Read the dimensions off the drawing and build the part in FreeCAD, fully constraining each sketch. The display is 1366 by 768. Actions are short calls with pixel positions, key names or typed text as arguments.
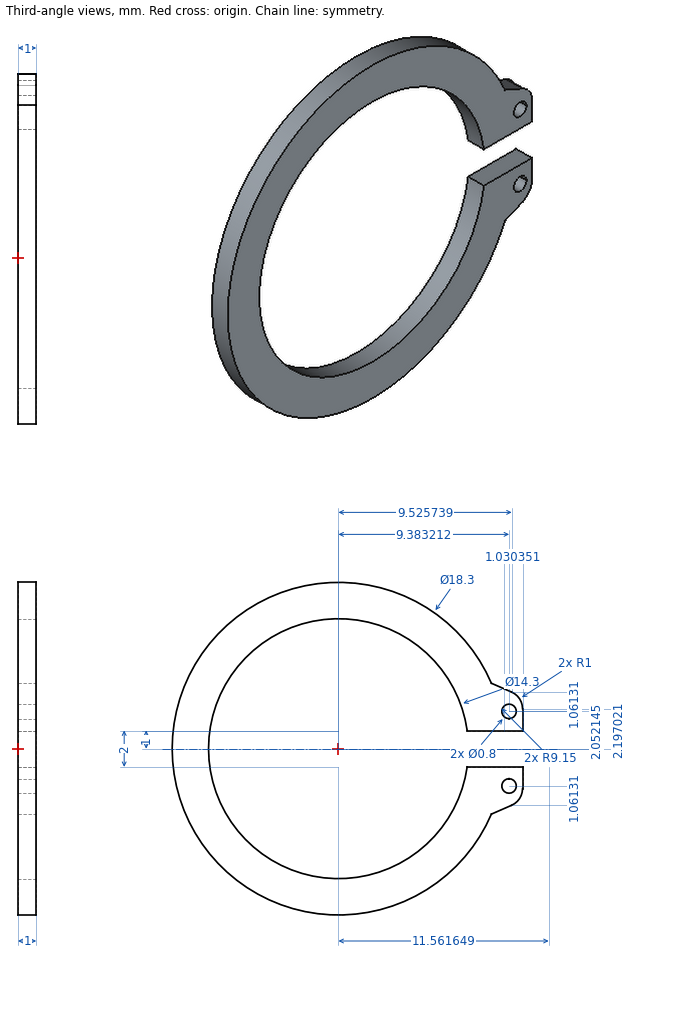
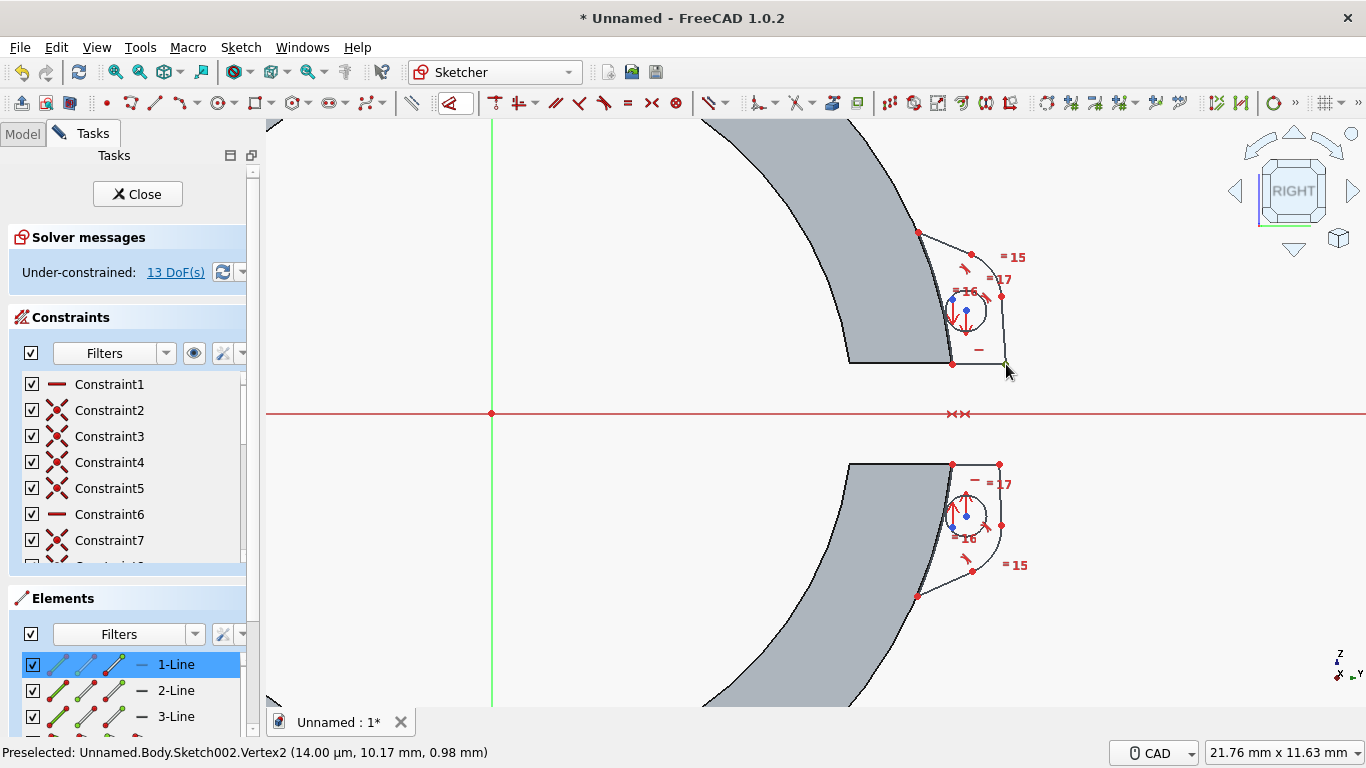
click(999, 465)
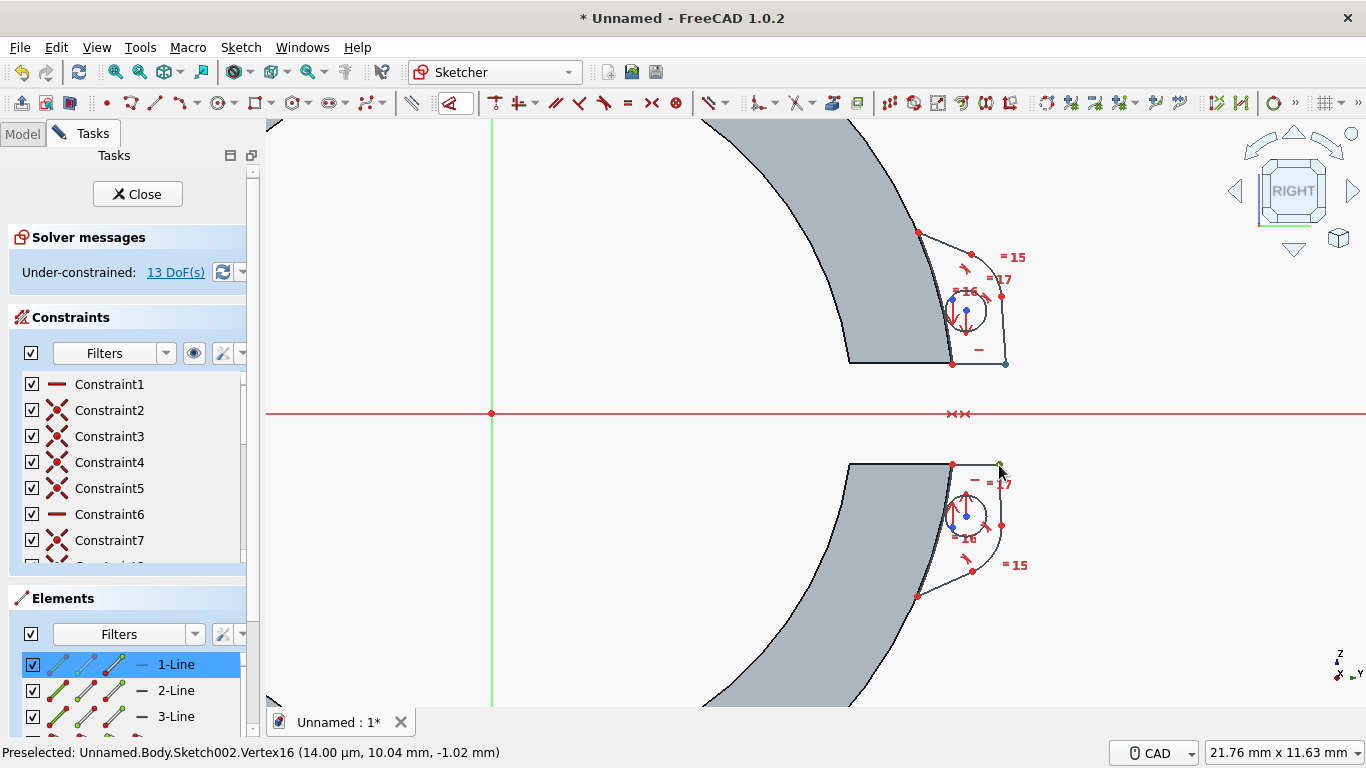
click(359, 414)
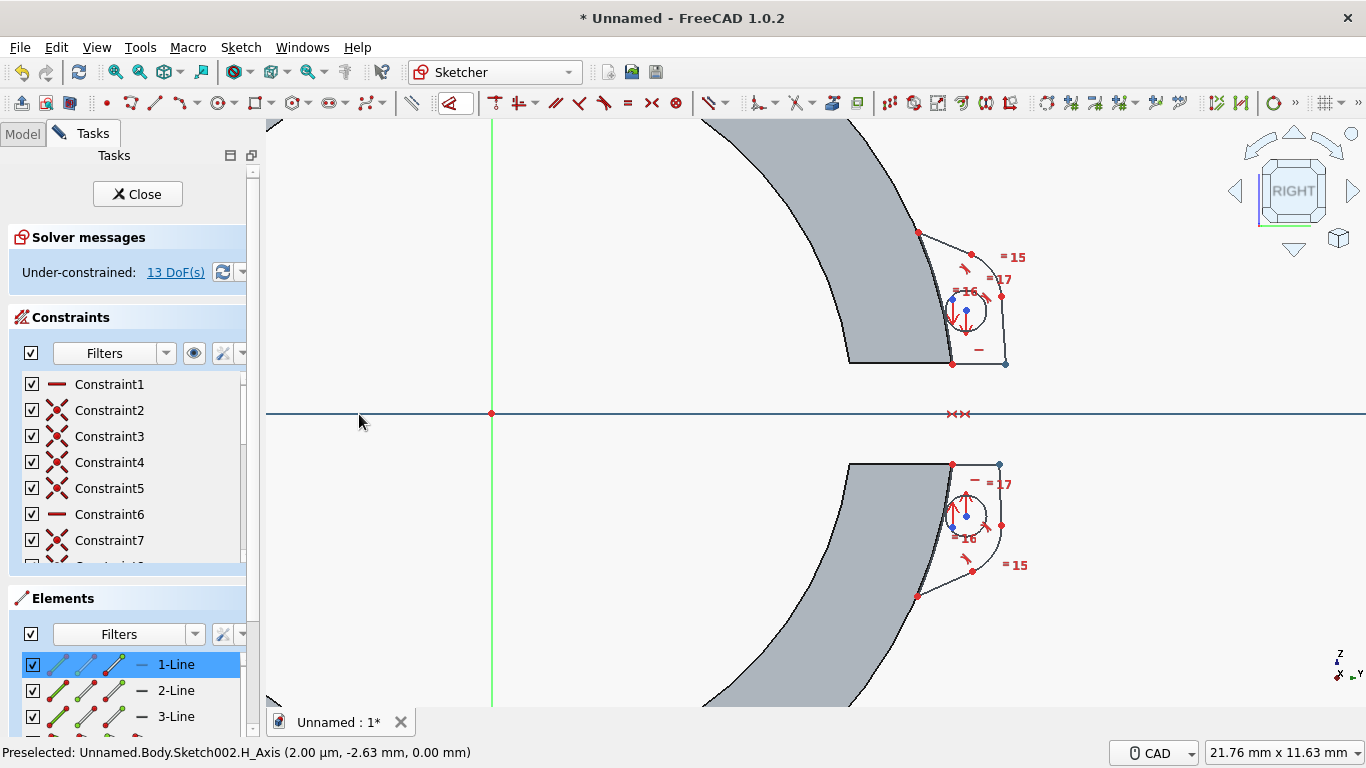
click(652, 104)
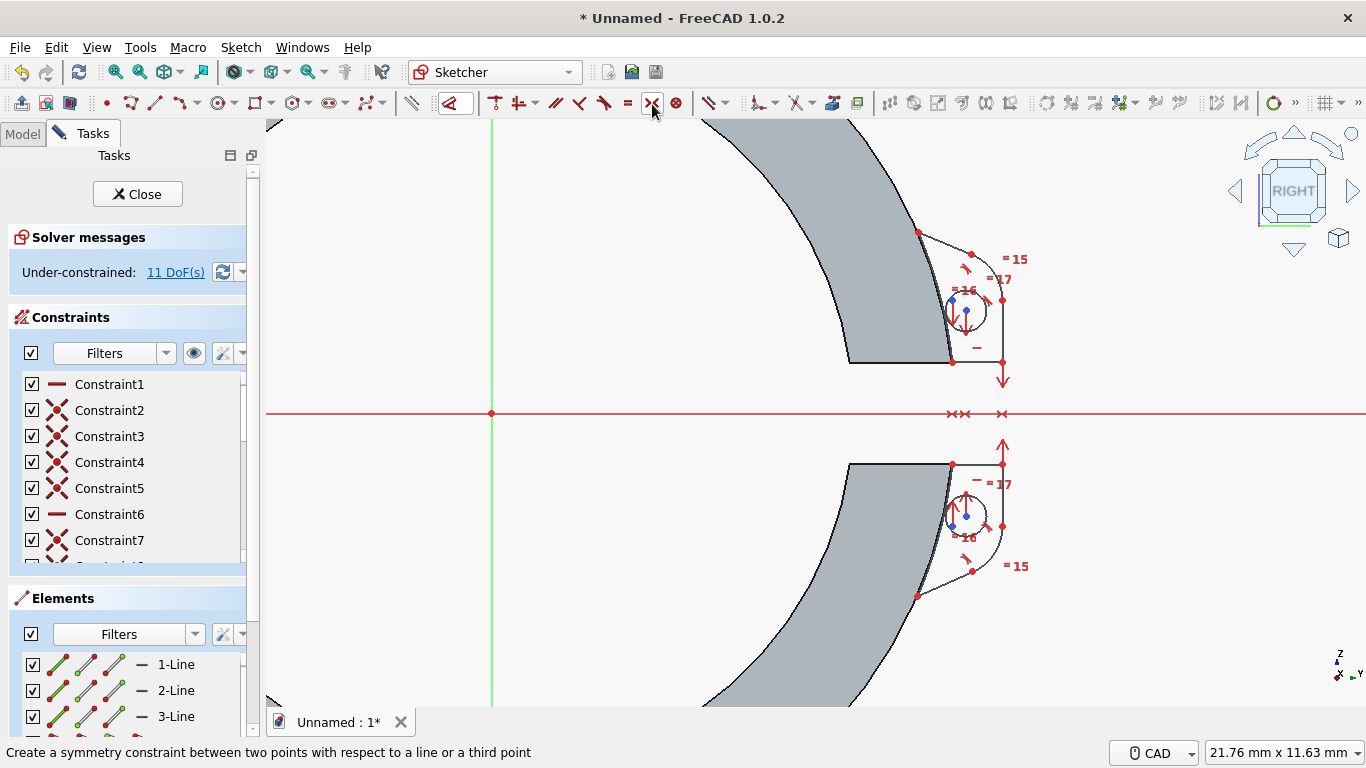
click(987, 264)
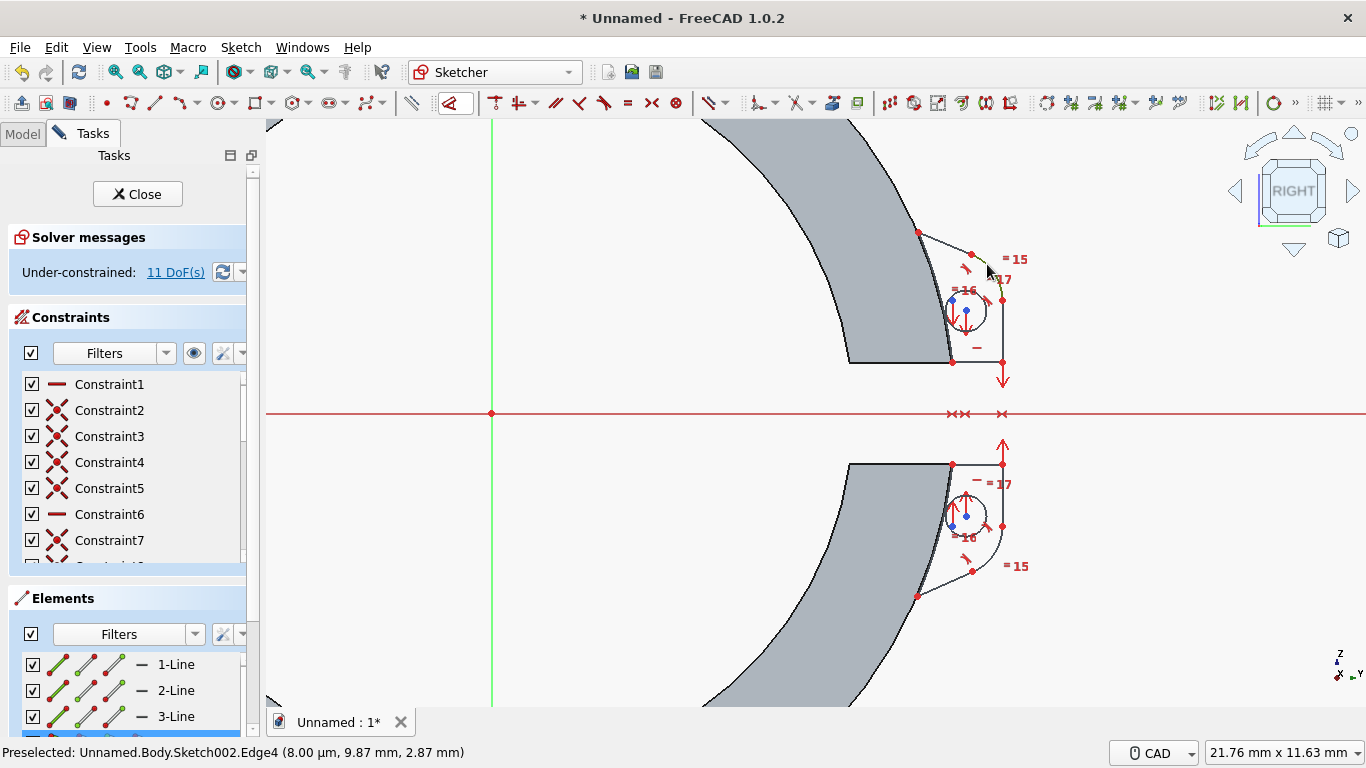
click(468, 104)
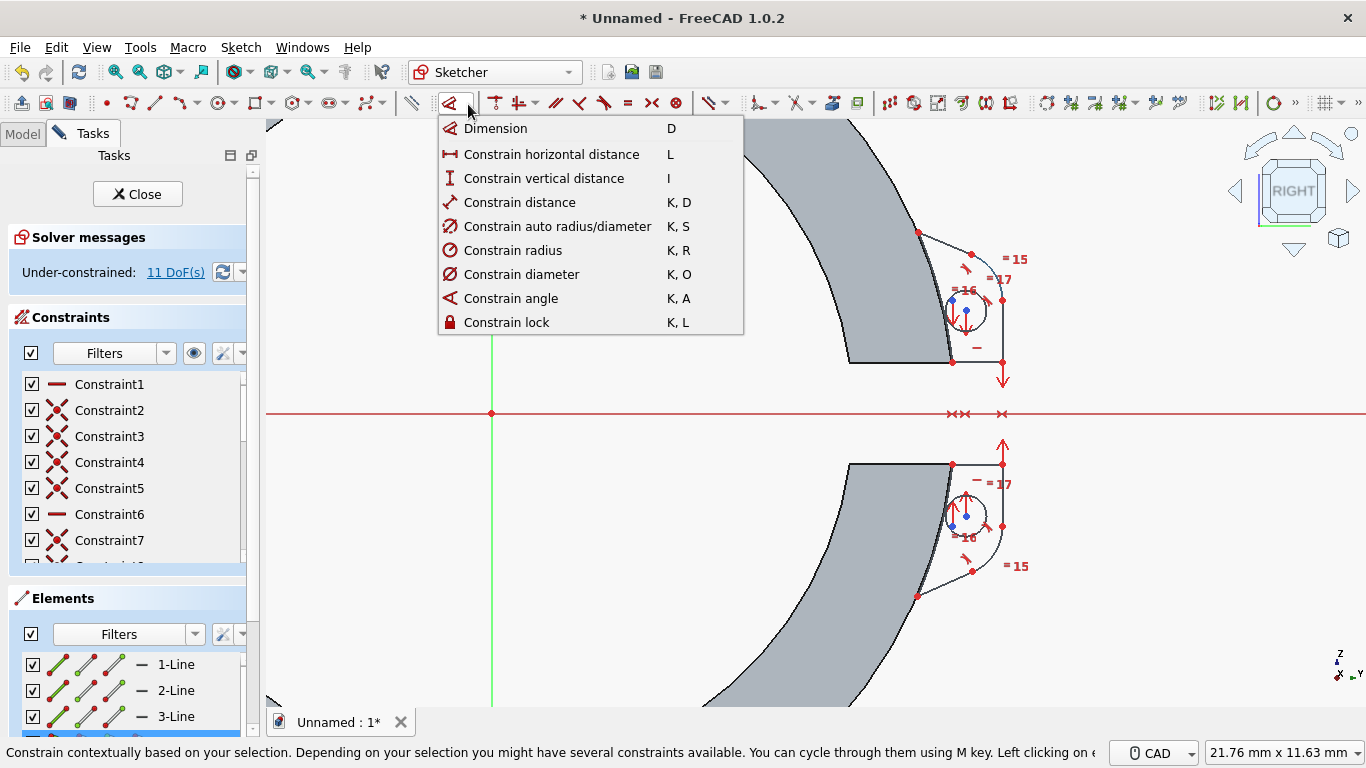
click(591, 250)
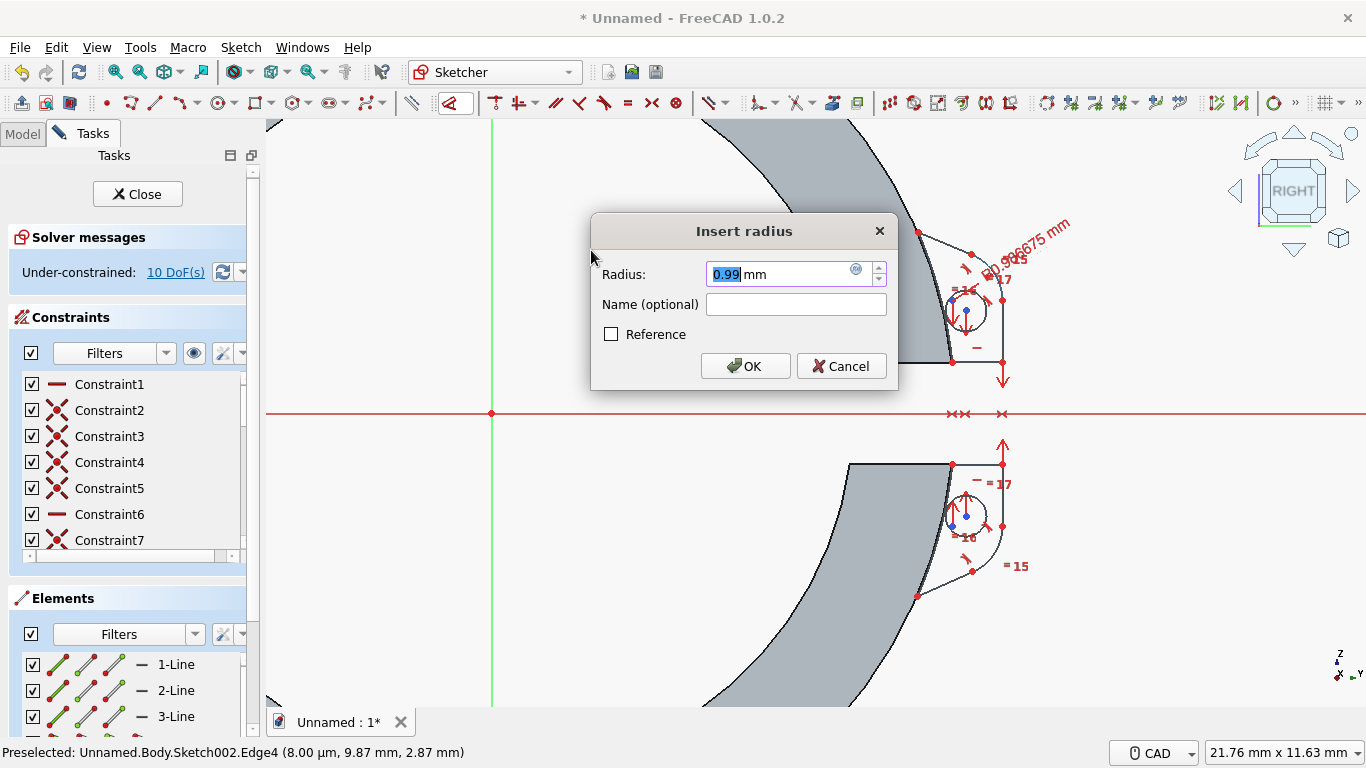
text(1)
key(Return)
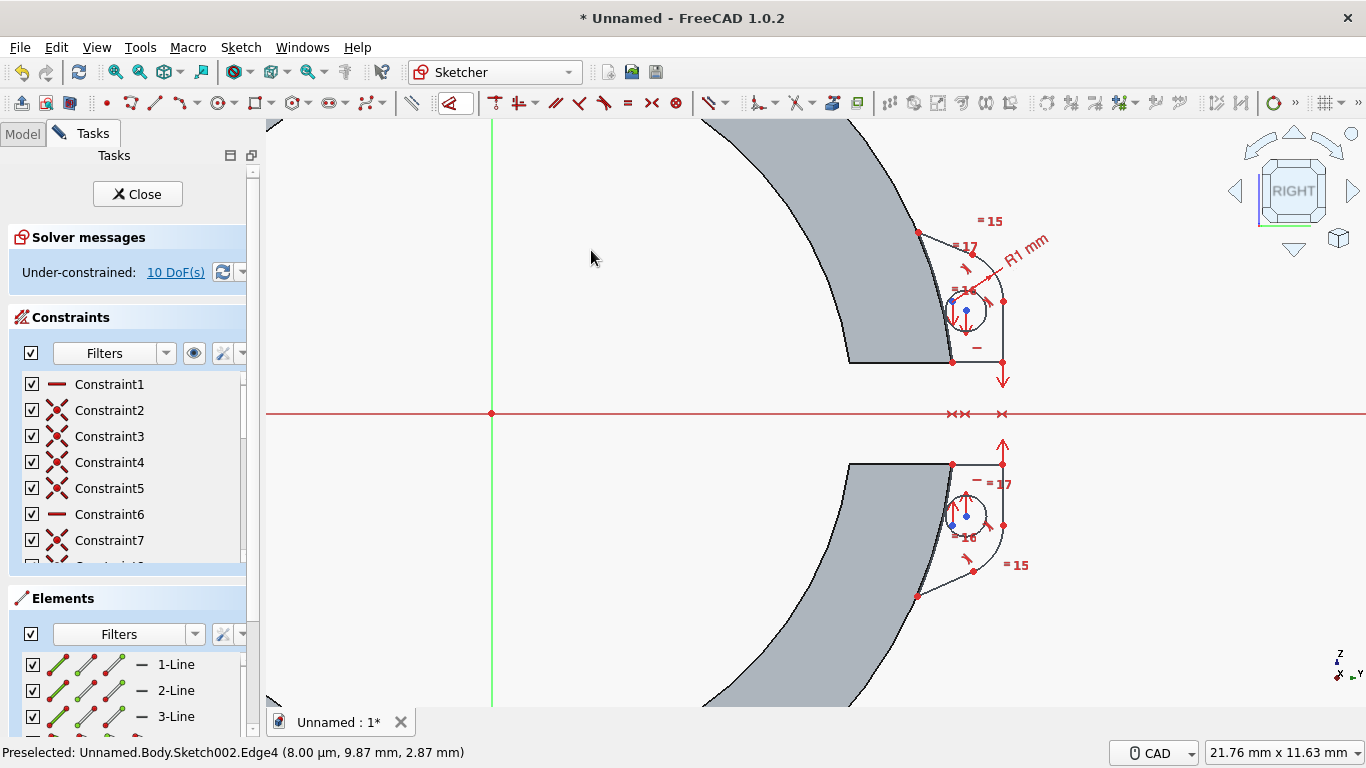
click(933, 270)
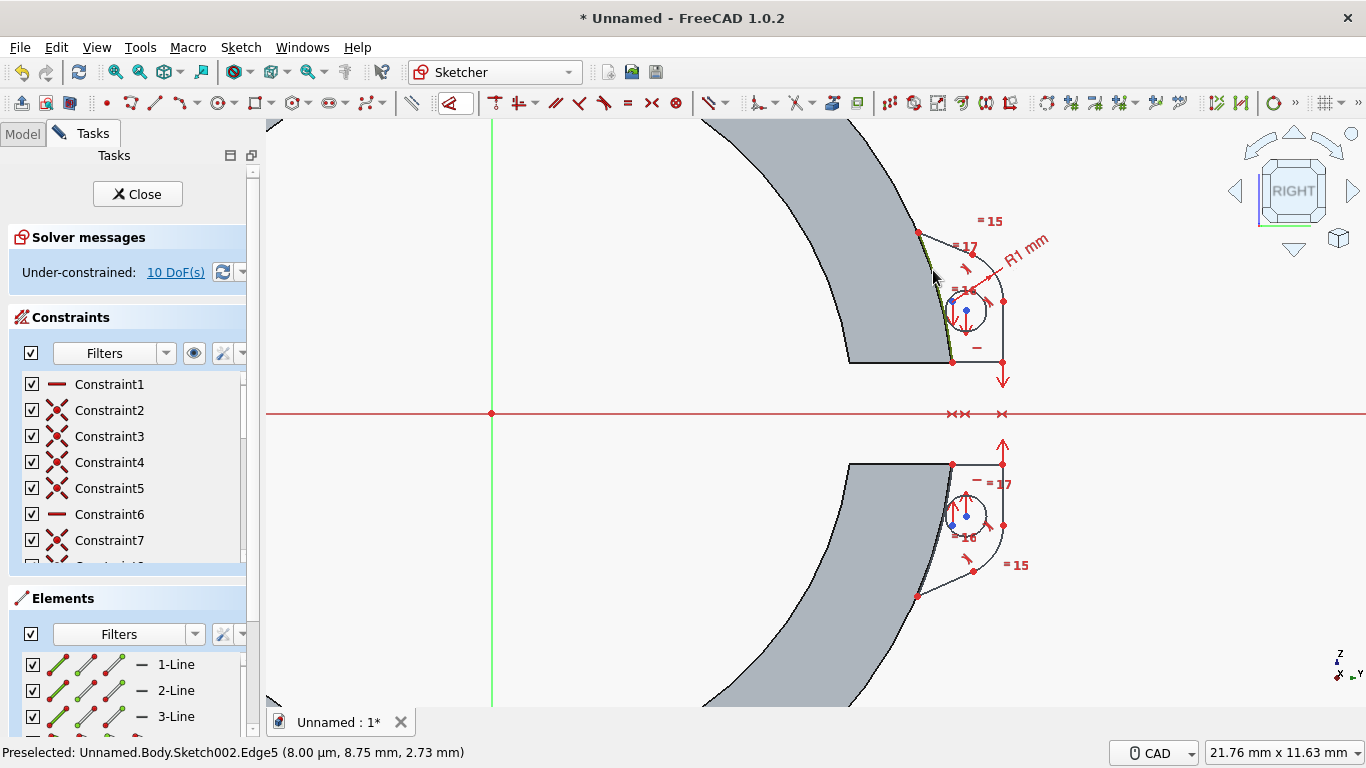
click(468, 104)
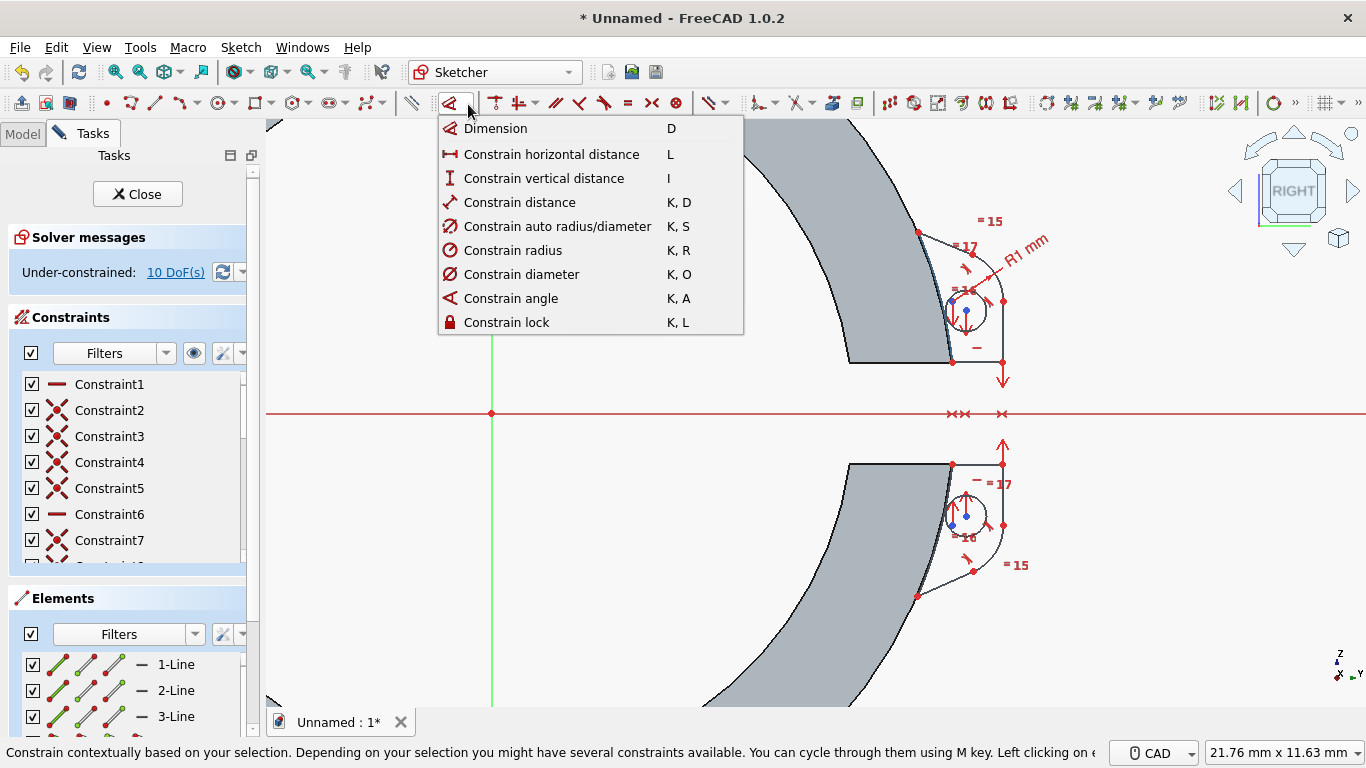
click(591, 250)